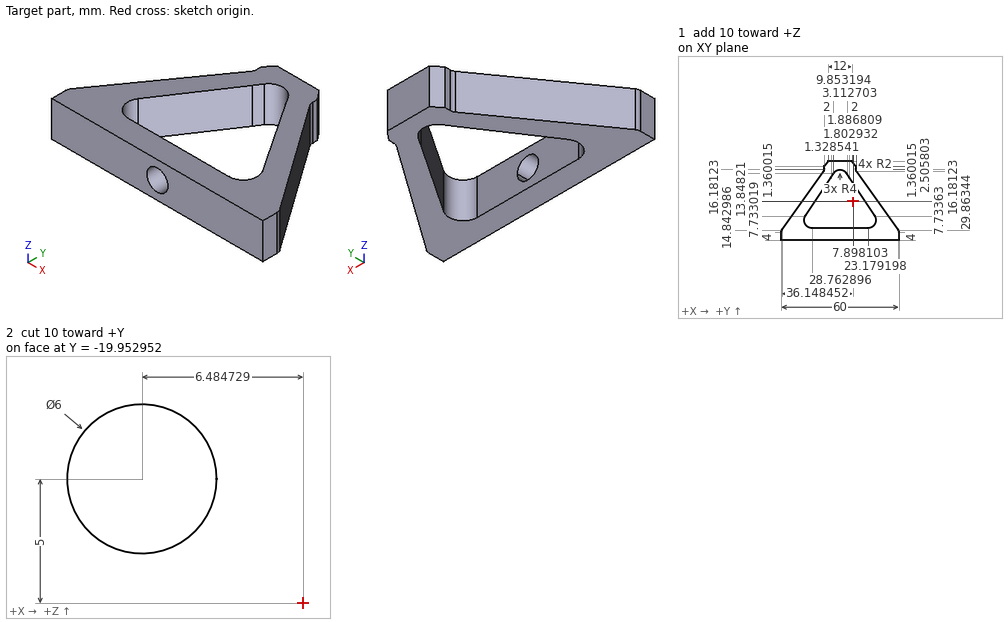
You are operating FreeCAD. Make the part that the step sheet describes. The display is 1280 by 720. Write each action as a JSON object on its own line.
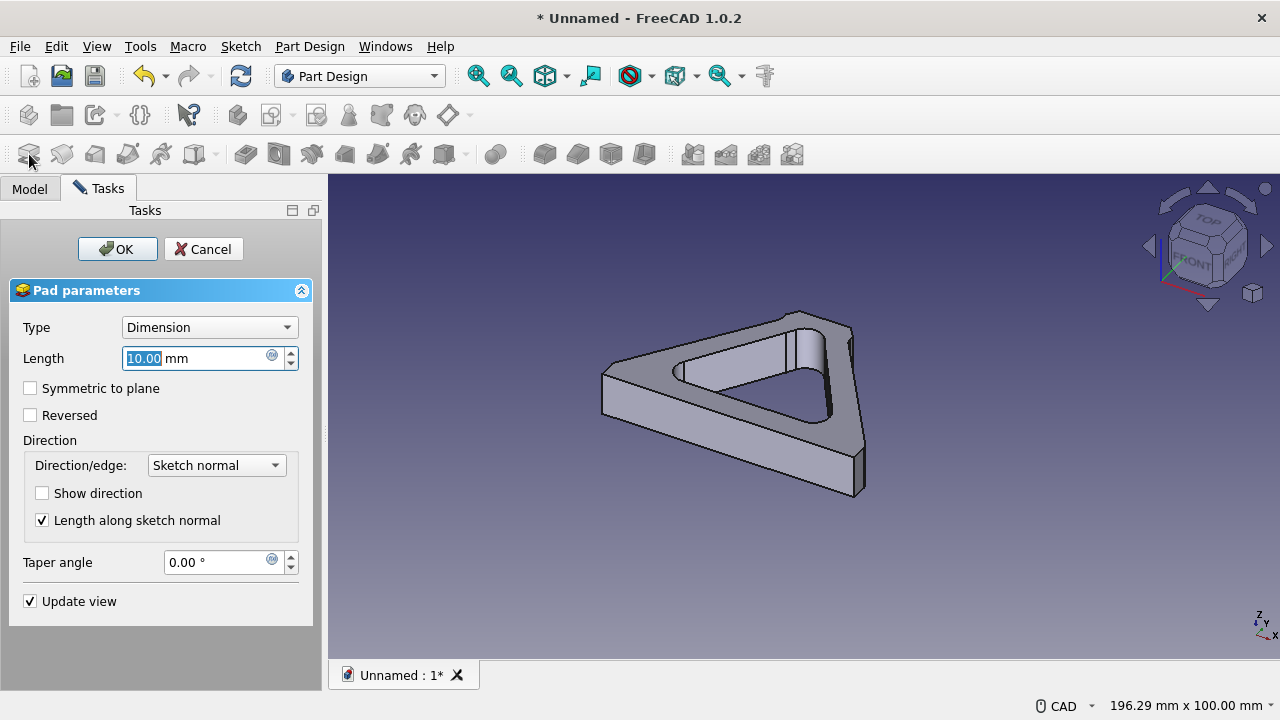
{"action": "type", "text": "10"}
{"action": "key", "text": "Tab"}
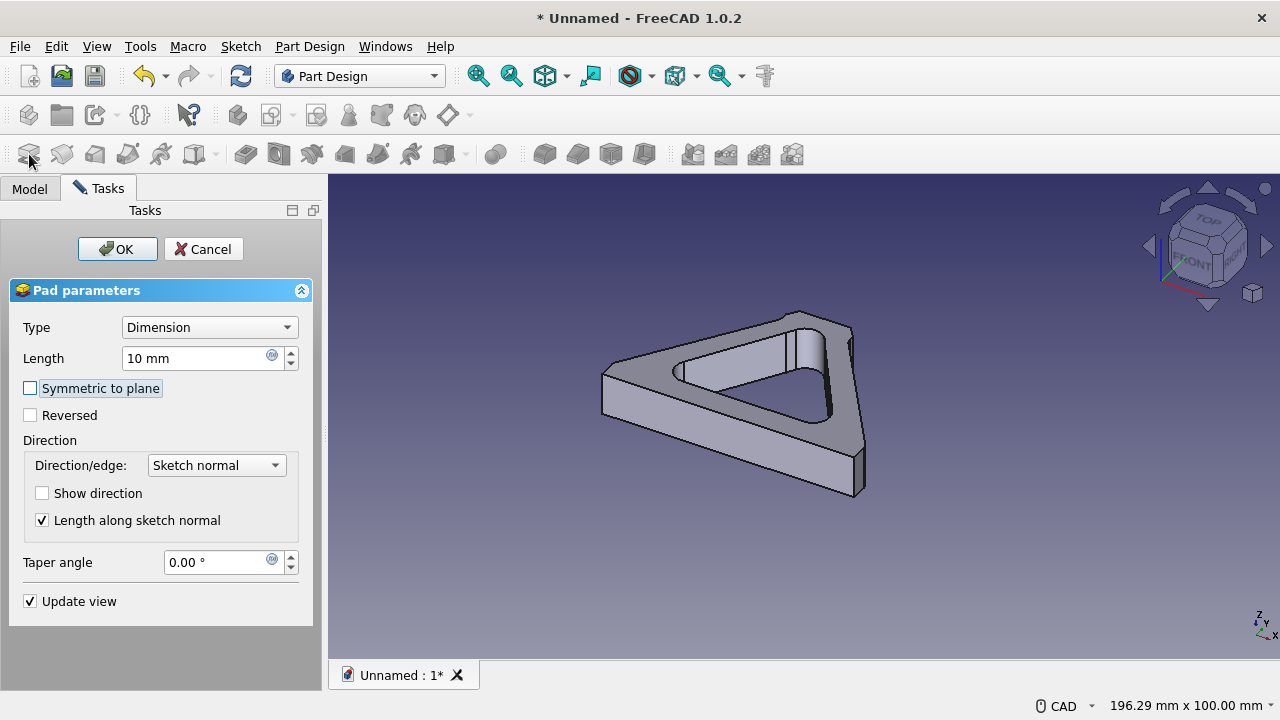
{"action": "left_click", "coordinate": [118, 249]}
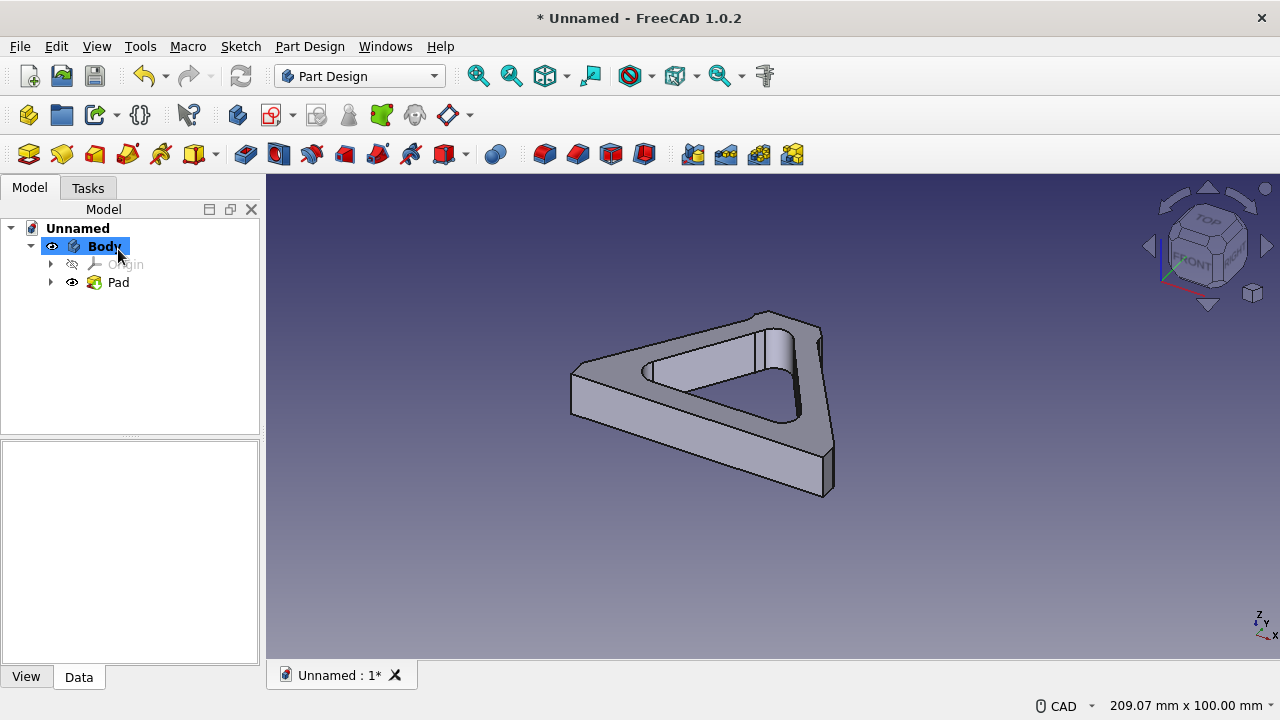
{"action": "left_click", "coordinate": [769, 459]}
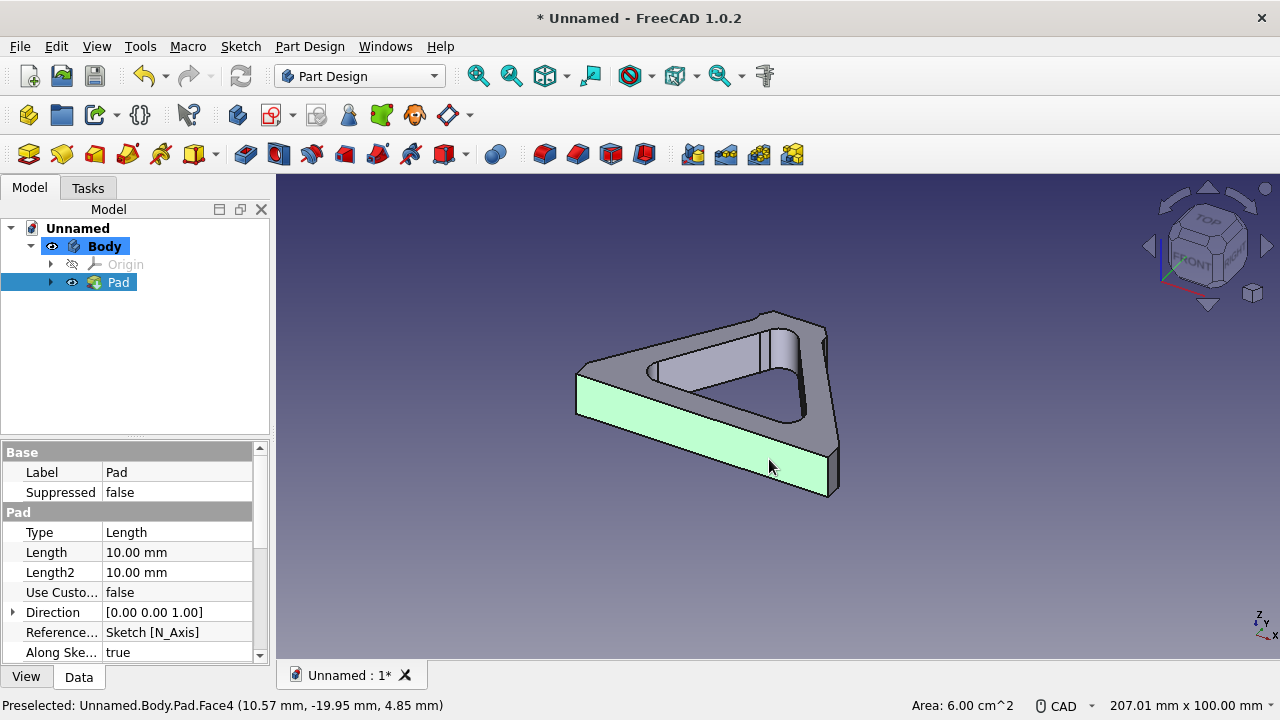
{"action": "left_click", "coordinate": [270, 116]}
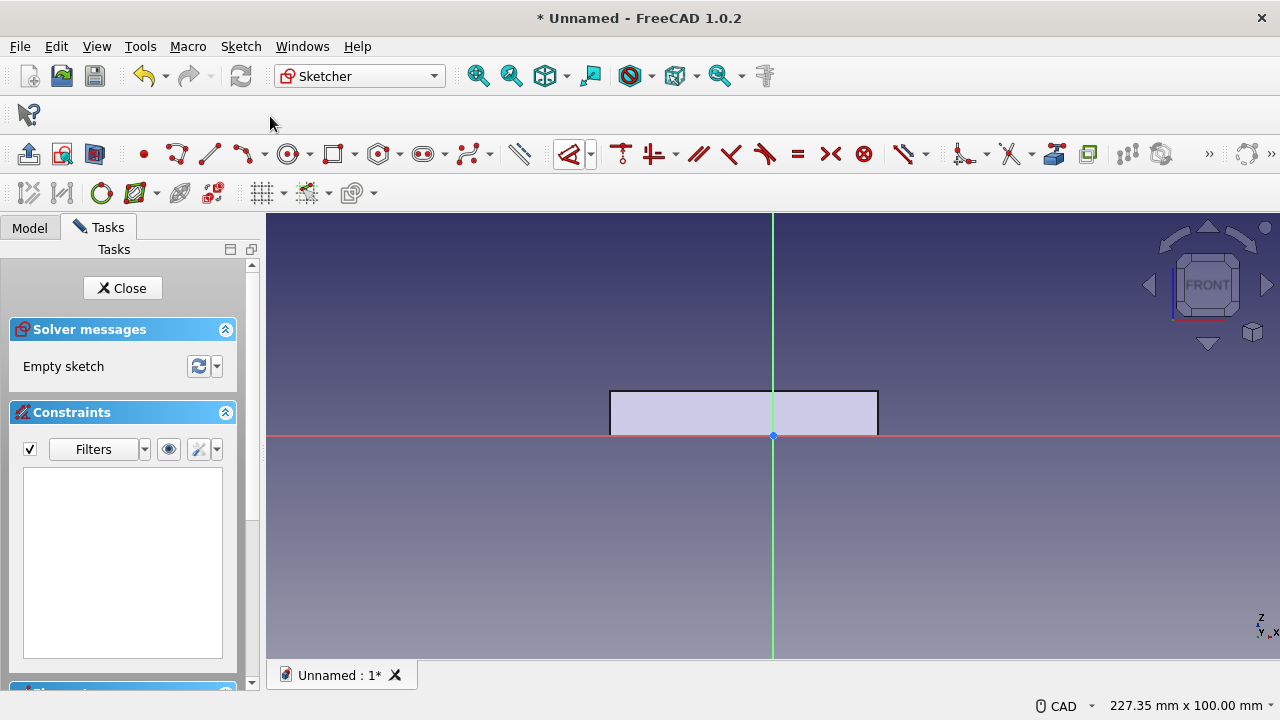
{"action": "scroll", "coordinate": [759, 415], "scroll_direction": "up", "scroll_amount": 10}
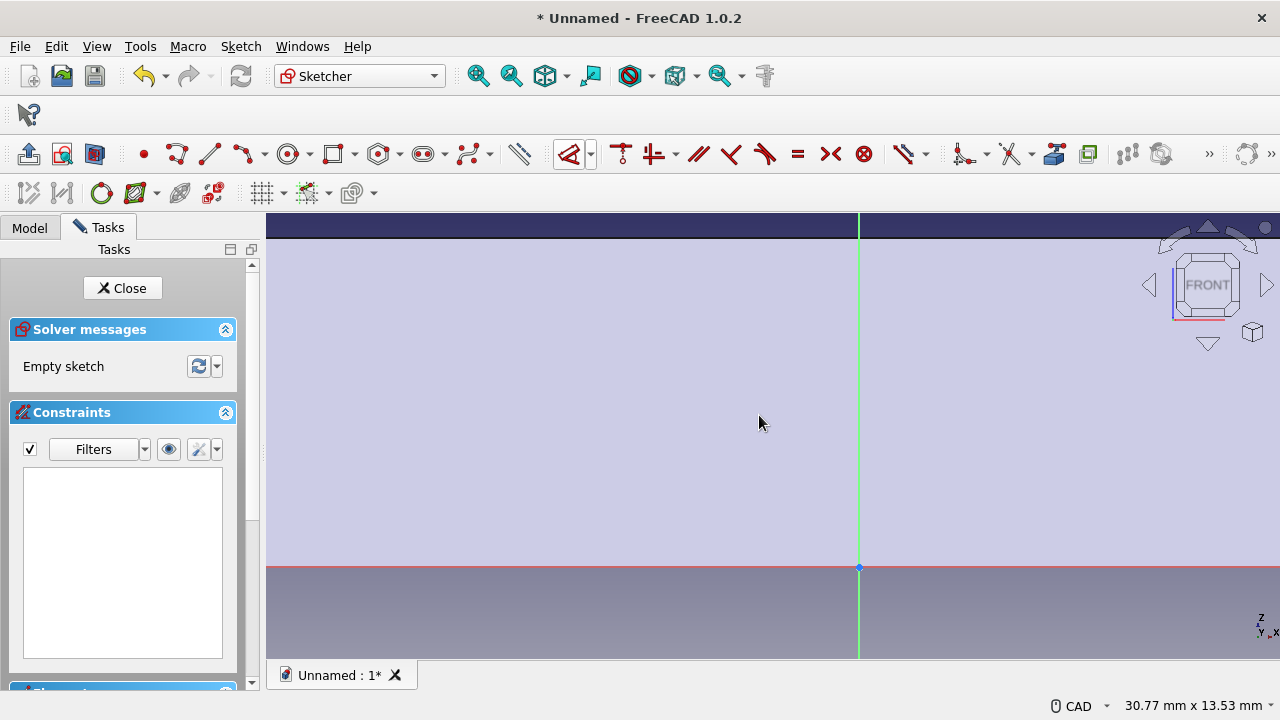
{"action": "left_click", "coordinate": [288, 154]}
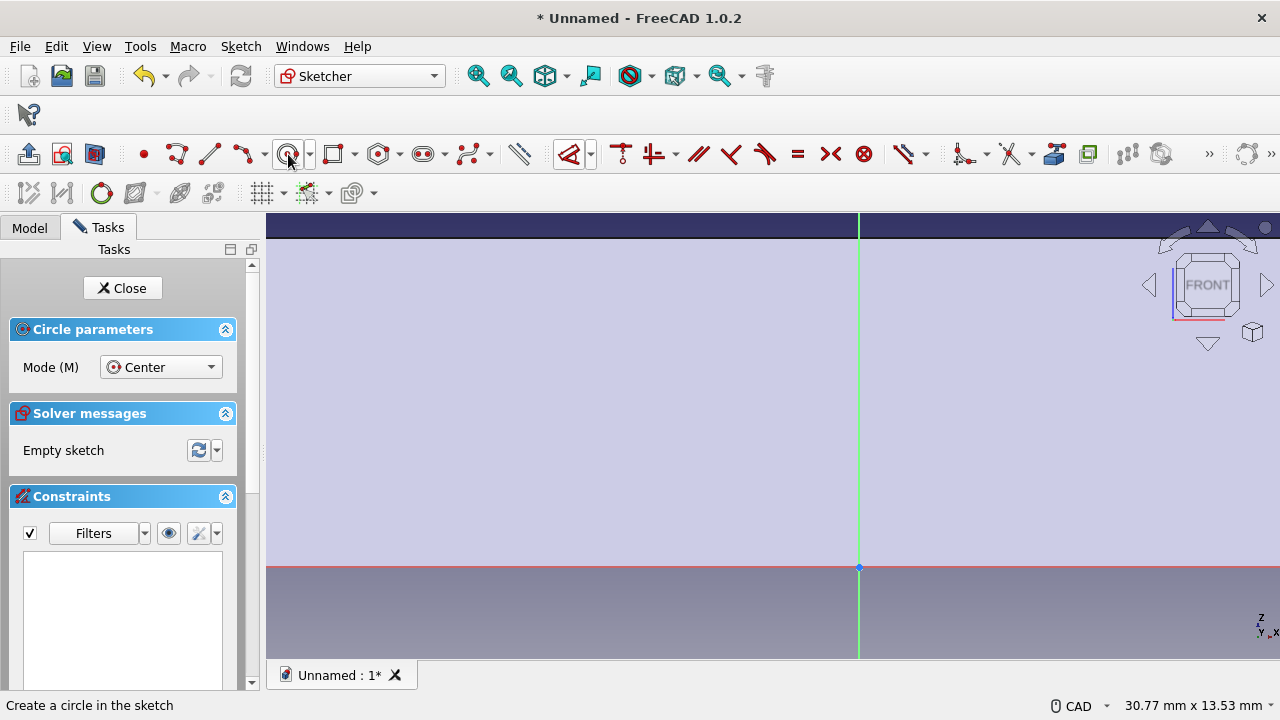
{"action": "left_click", "coordinate": [646, 402]}
{"action": "left_click", "coordinate": [716, 333]}
{"action": "key", "text": "Escape"}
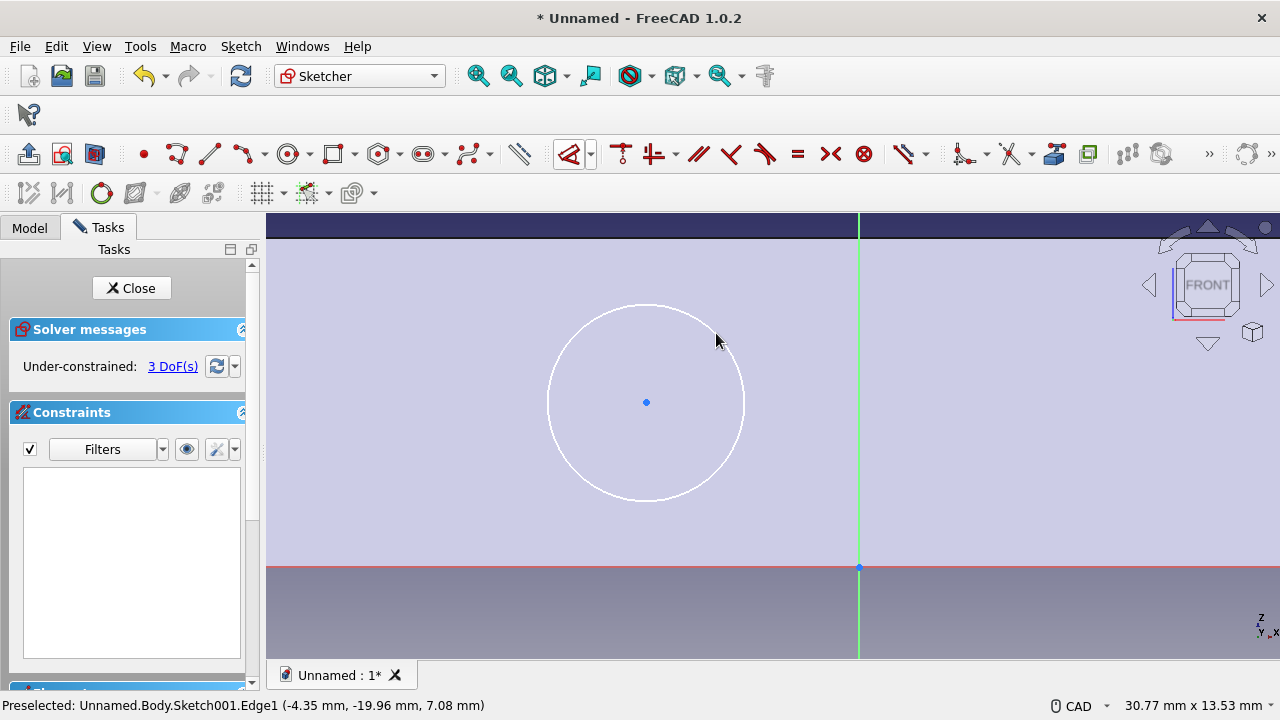
{"action": "left_click", "coordinate": [715, 333]}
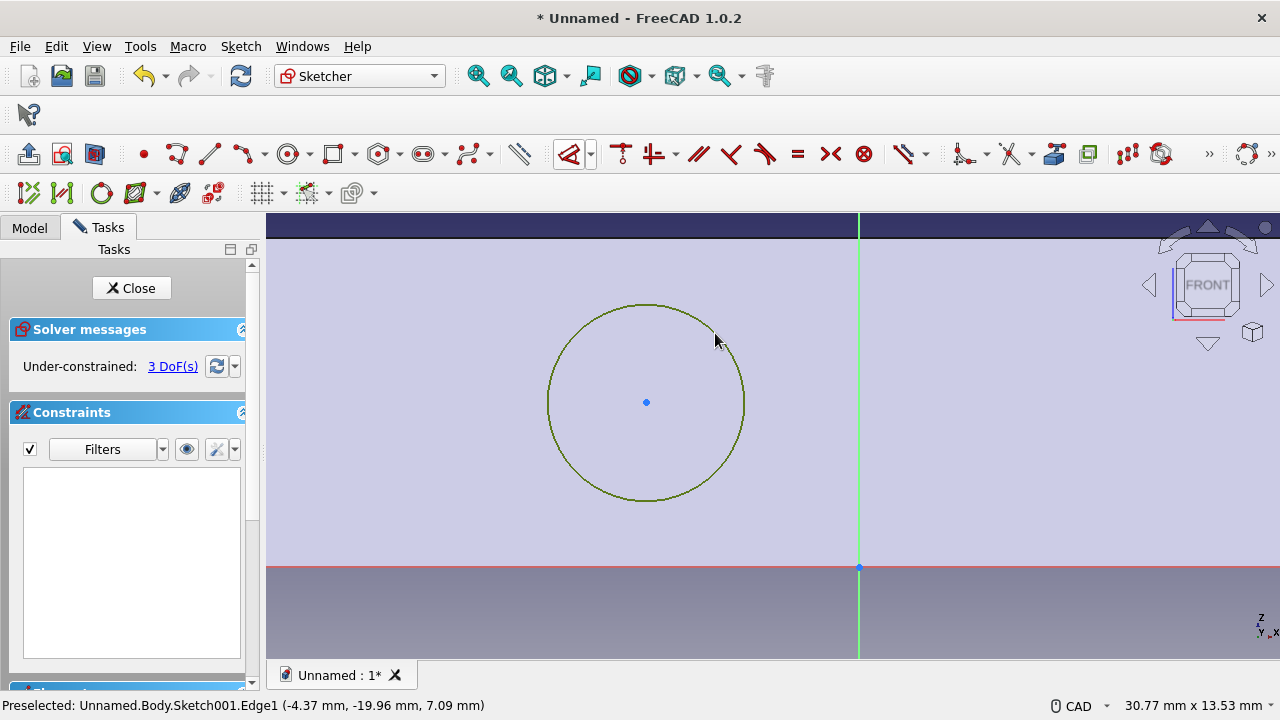
{"action": "left_click", "coordinate": [590, 154]}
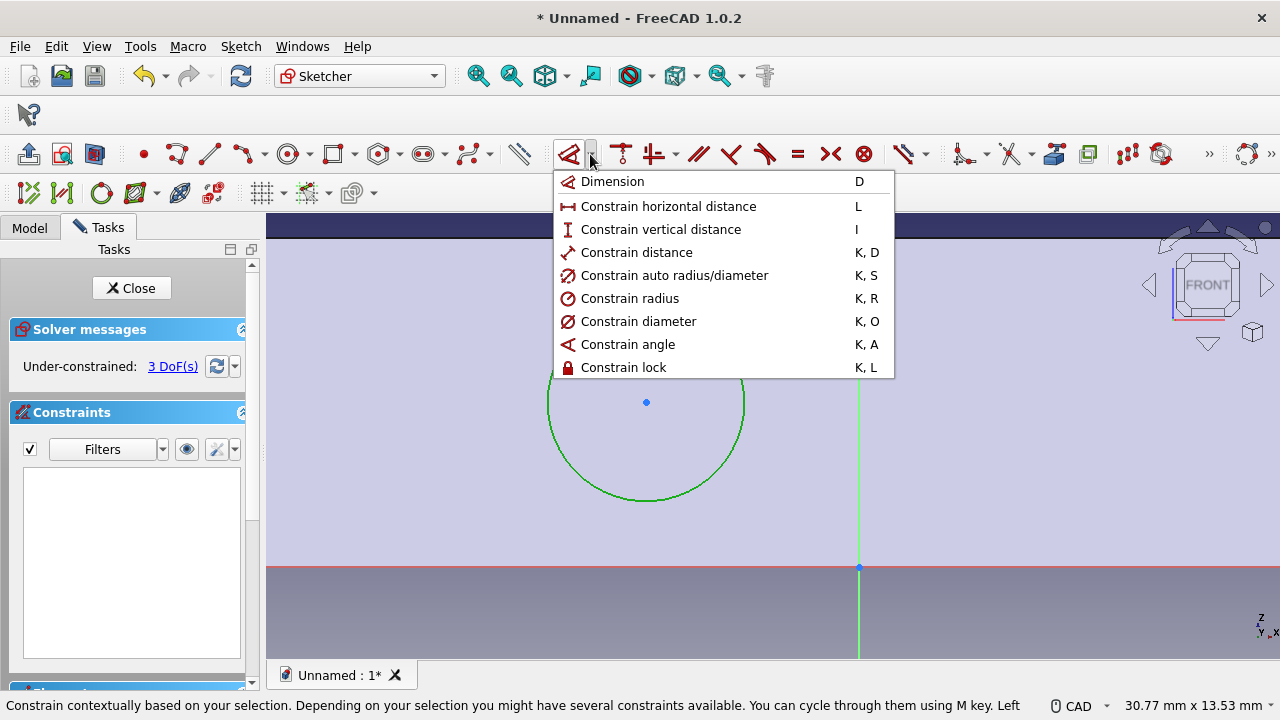
{"action": "left_click", "coordinate": [724, 322]}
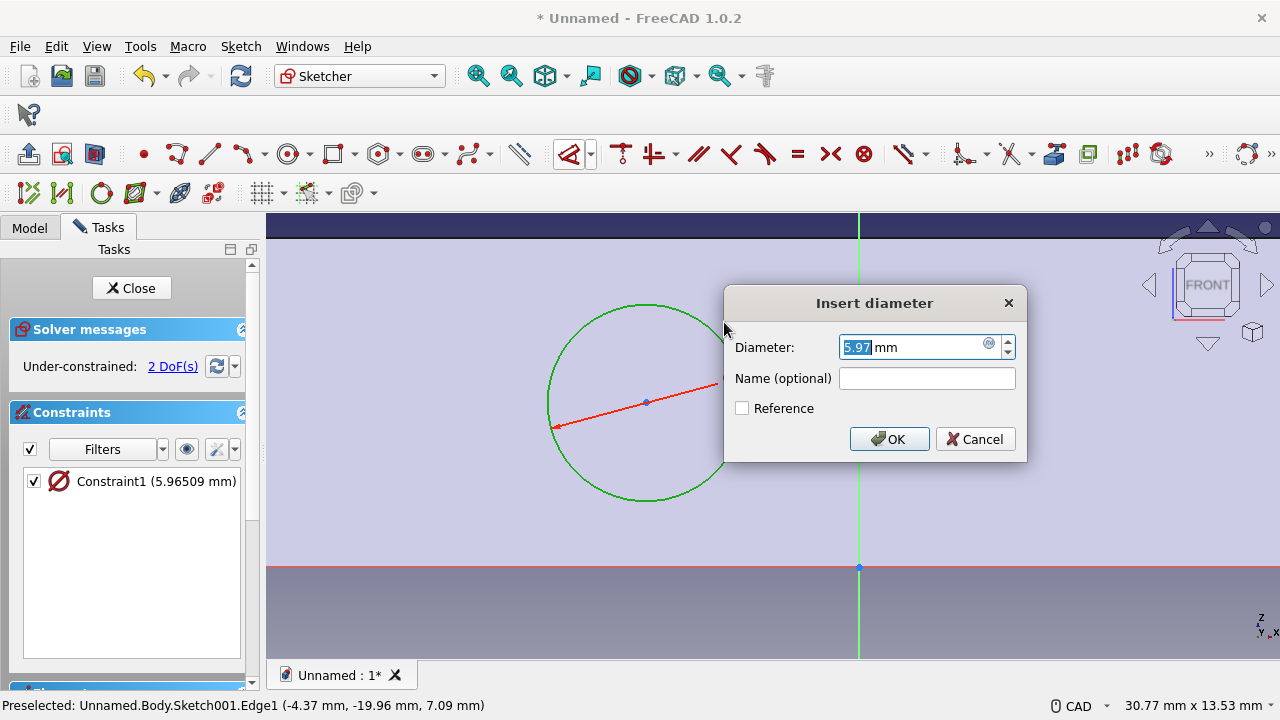
{"action": "type", "text": "6"}
{"action": "key", "text": "Return"}